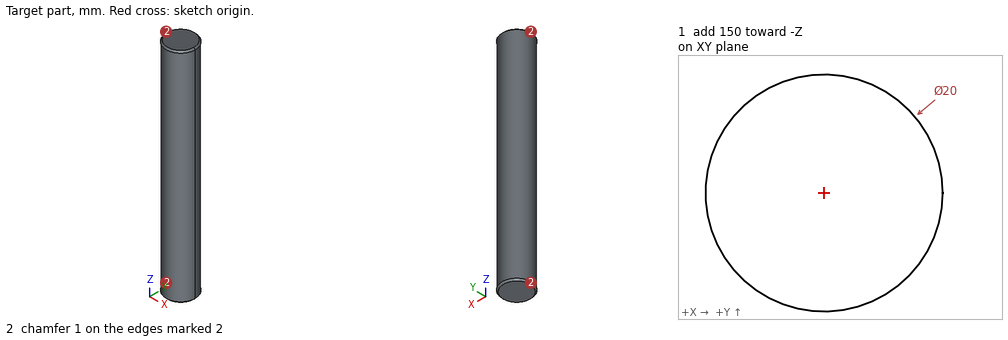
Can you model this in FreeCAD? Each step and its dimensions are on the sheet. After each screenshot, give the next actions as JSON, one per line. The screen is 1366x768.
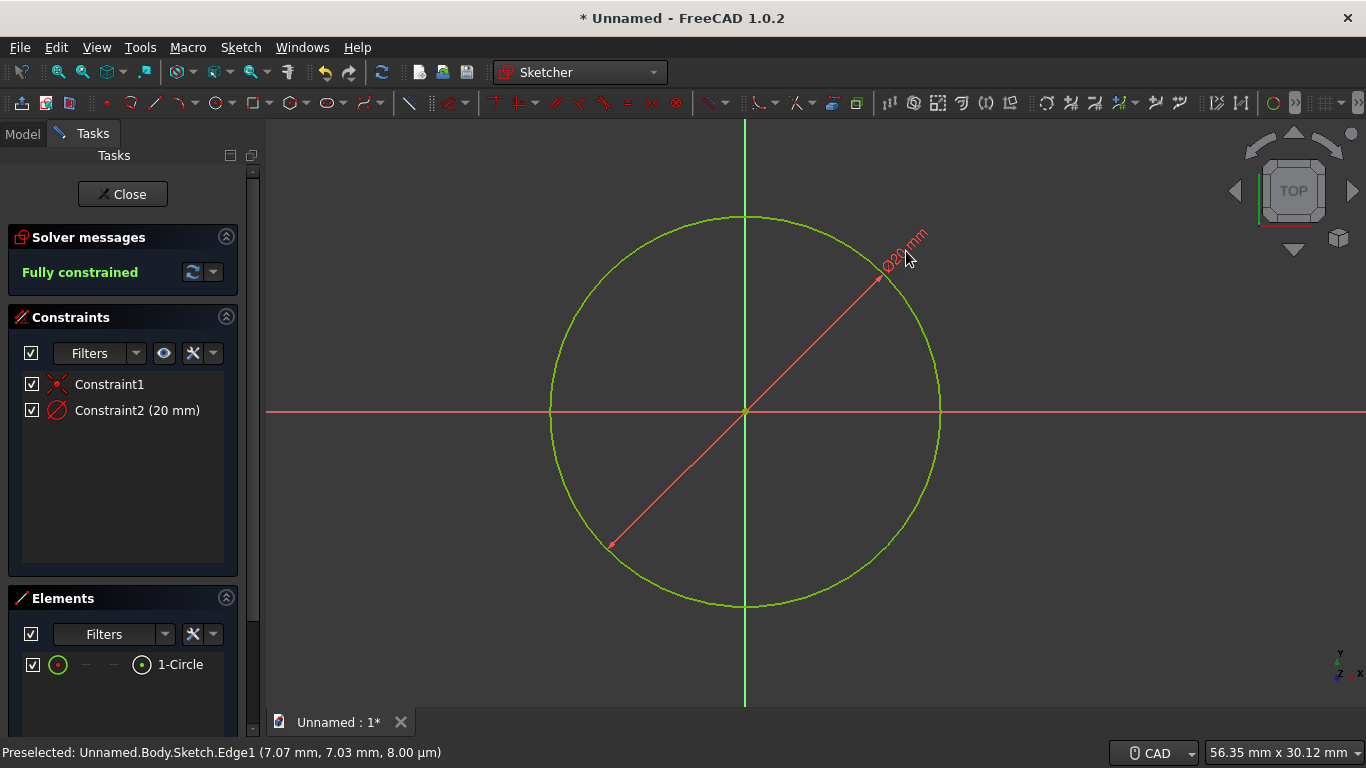
{"action": "left_click", "coordinate": [123, 194]}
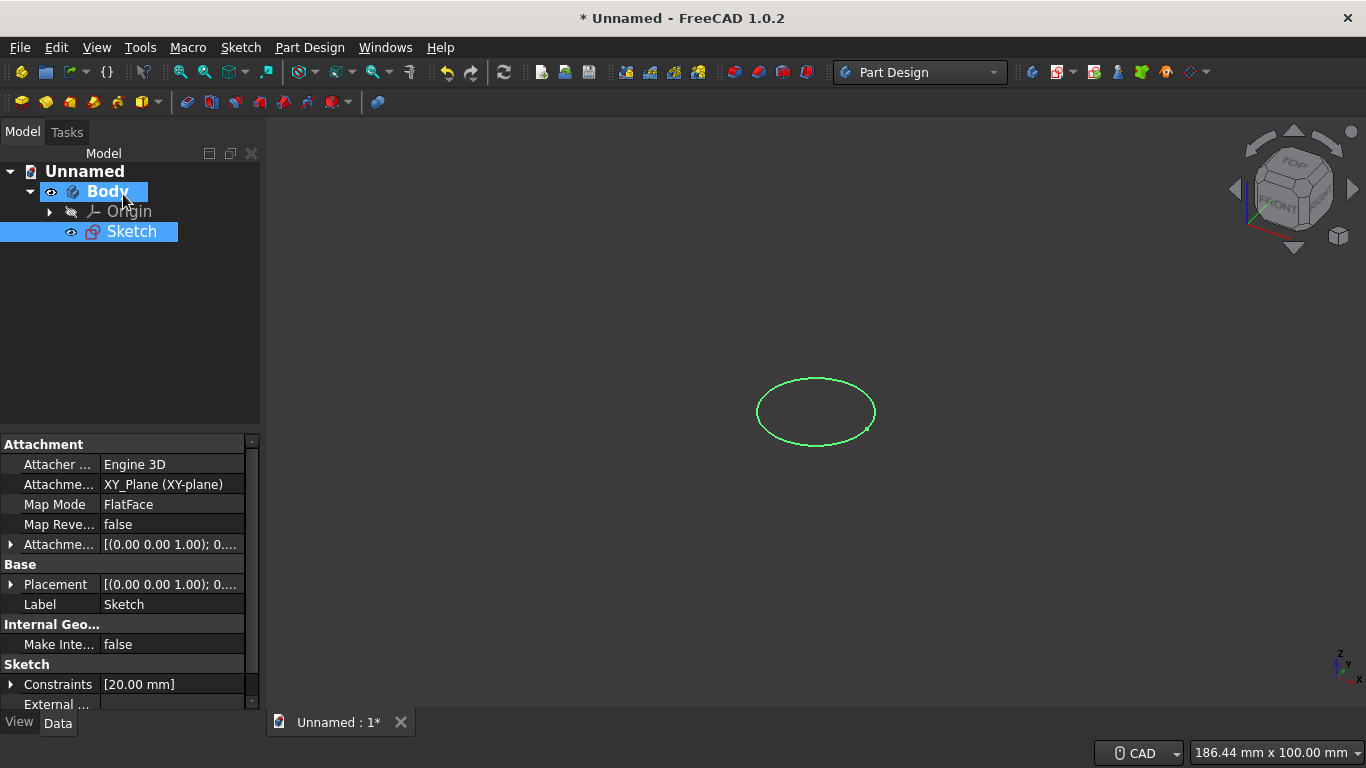
{"action": "left_click", "coordinate": [22, 102]}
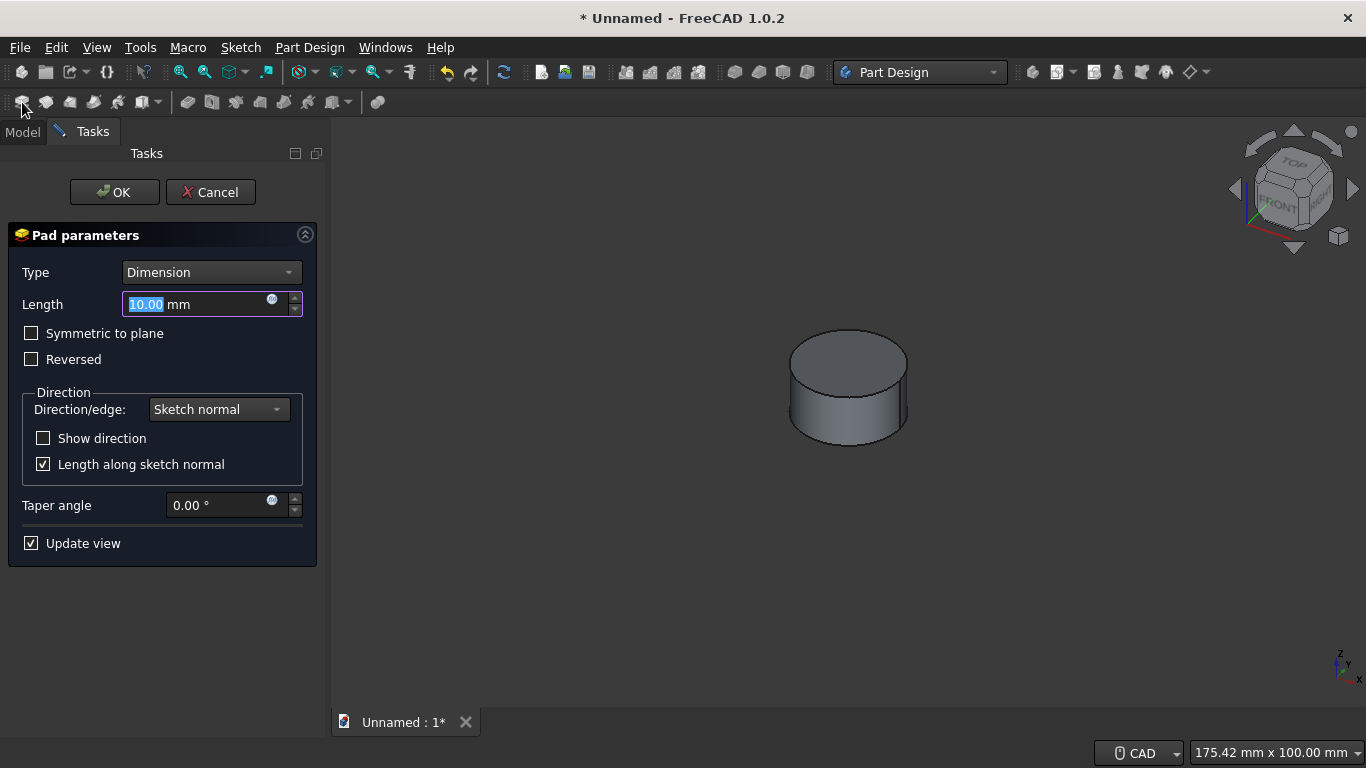
{"action": "type", "text": "150"}
{"action": "key", "text": "Tab"}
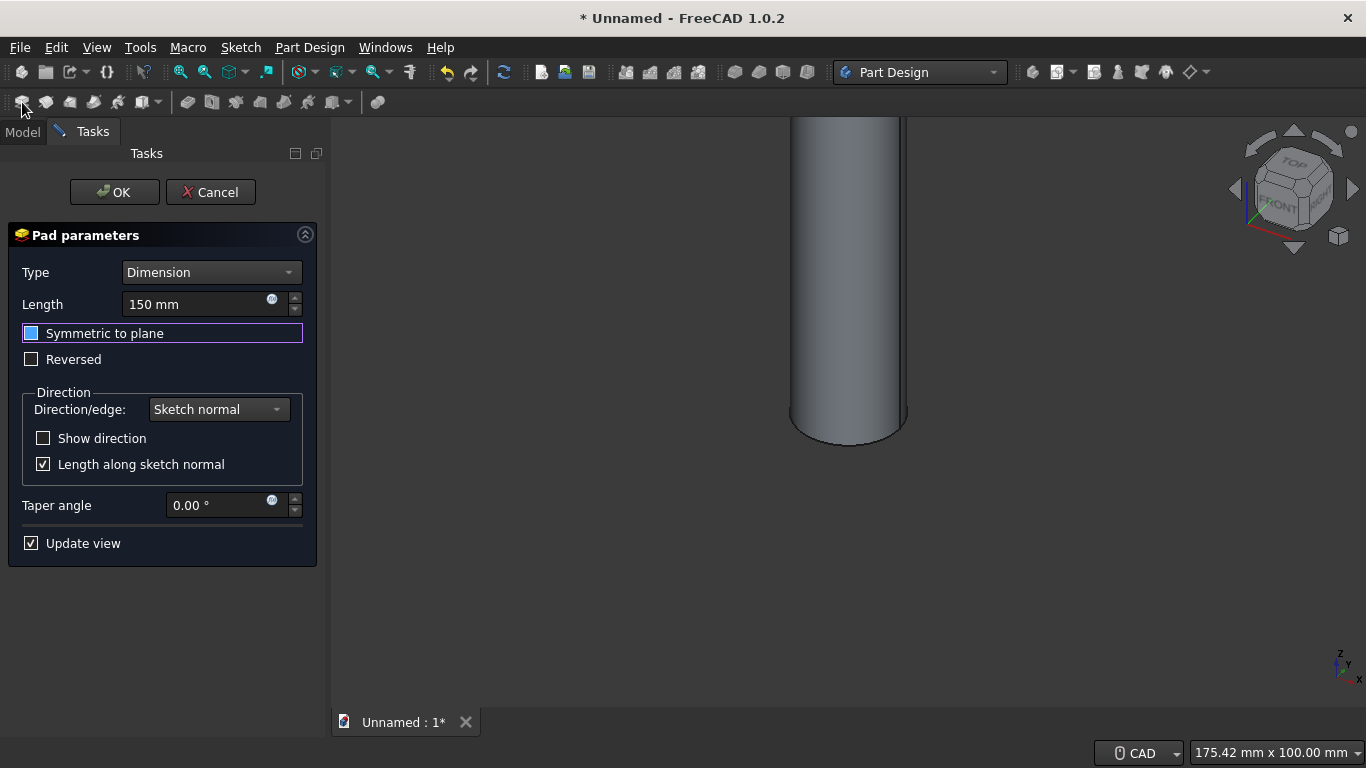
{"action": "left_click", "coordinate": [30, 359]}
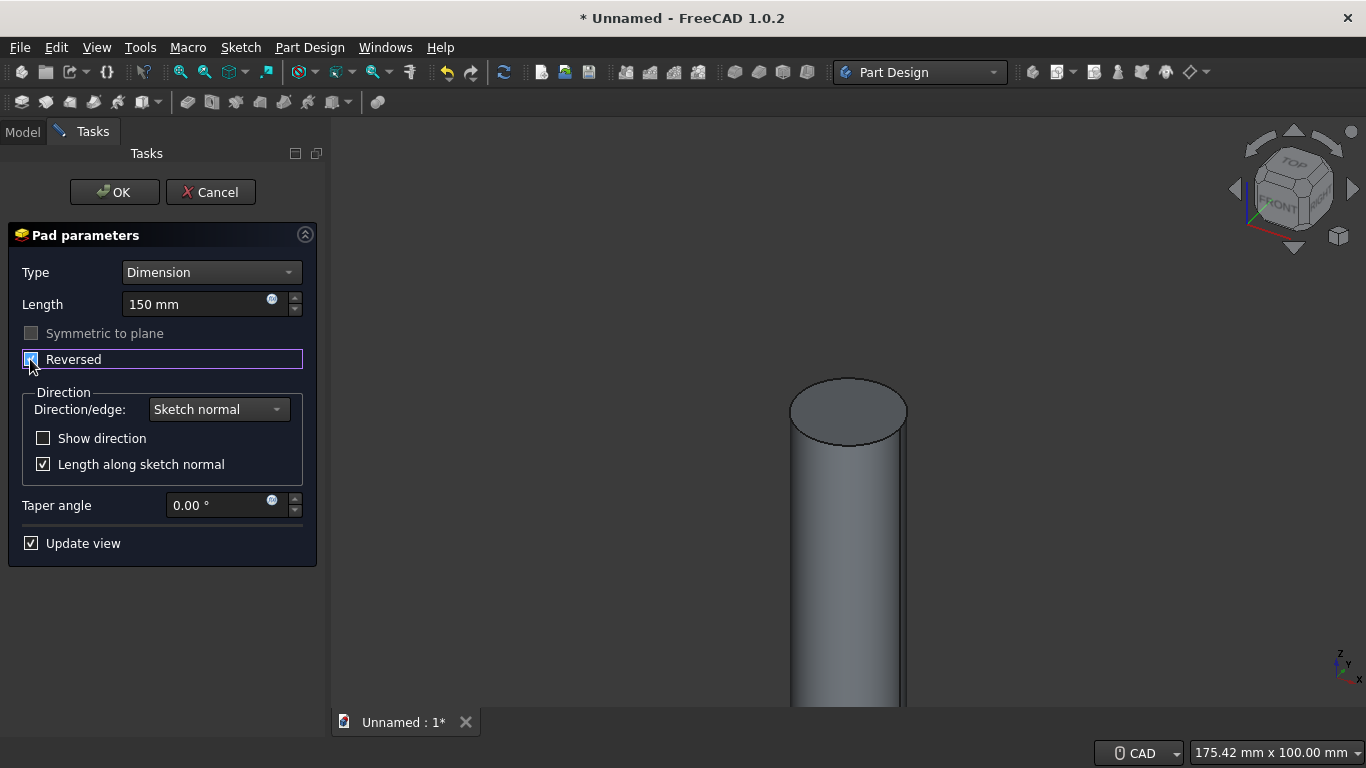
{"action": "left_click", "coordinate": [115, 192]}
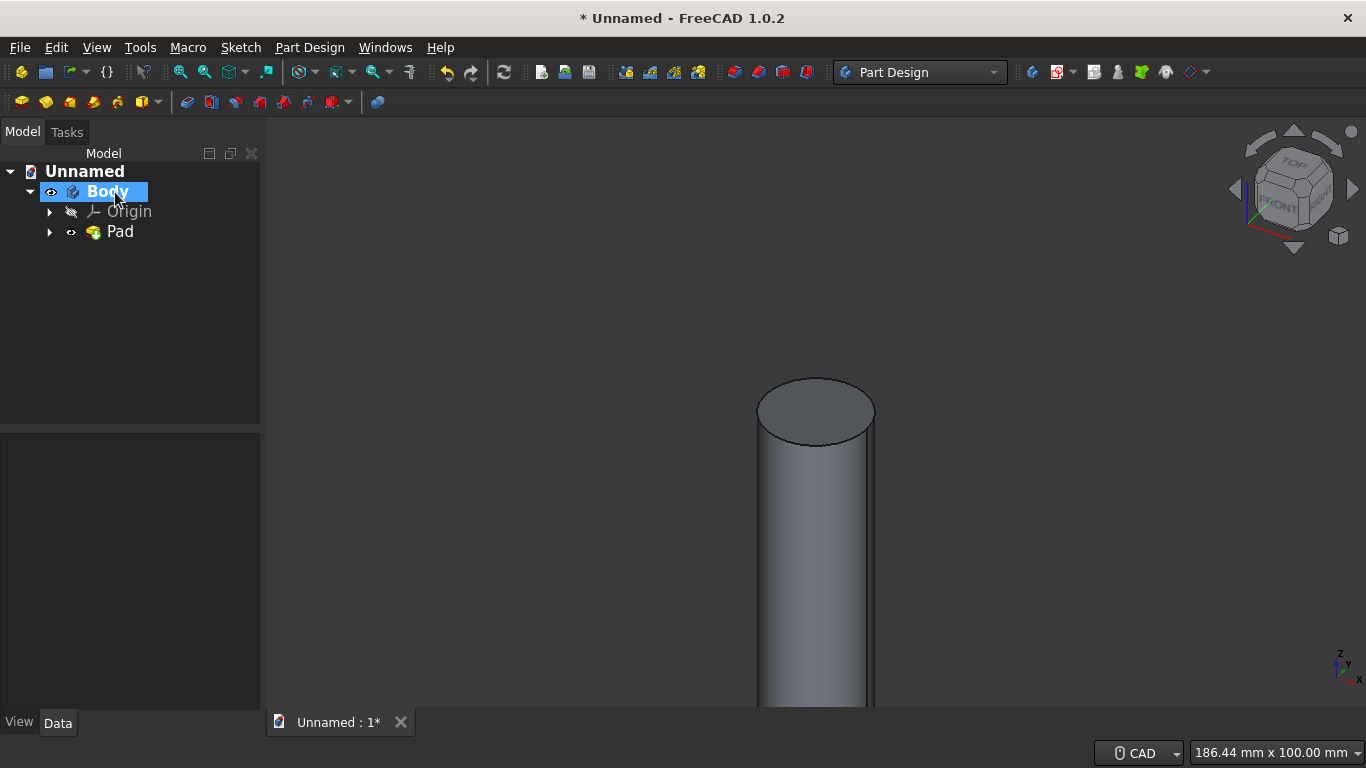
{"action": "key", "text": "v f"}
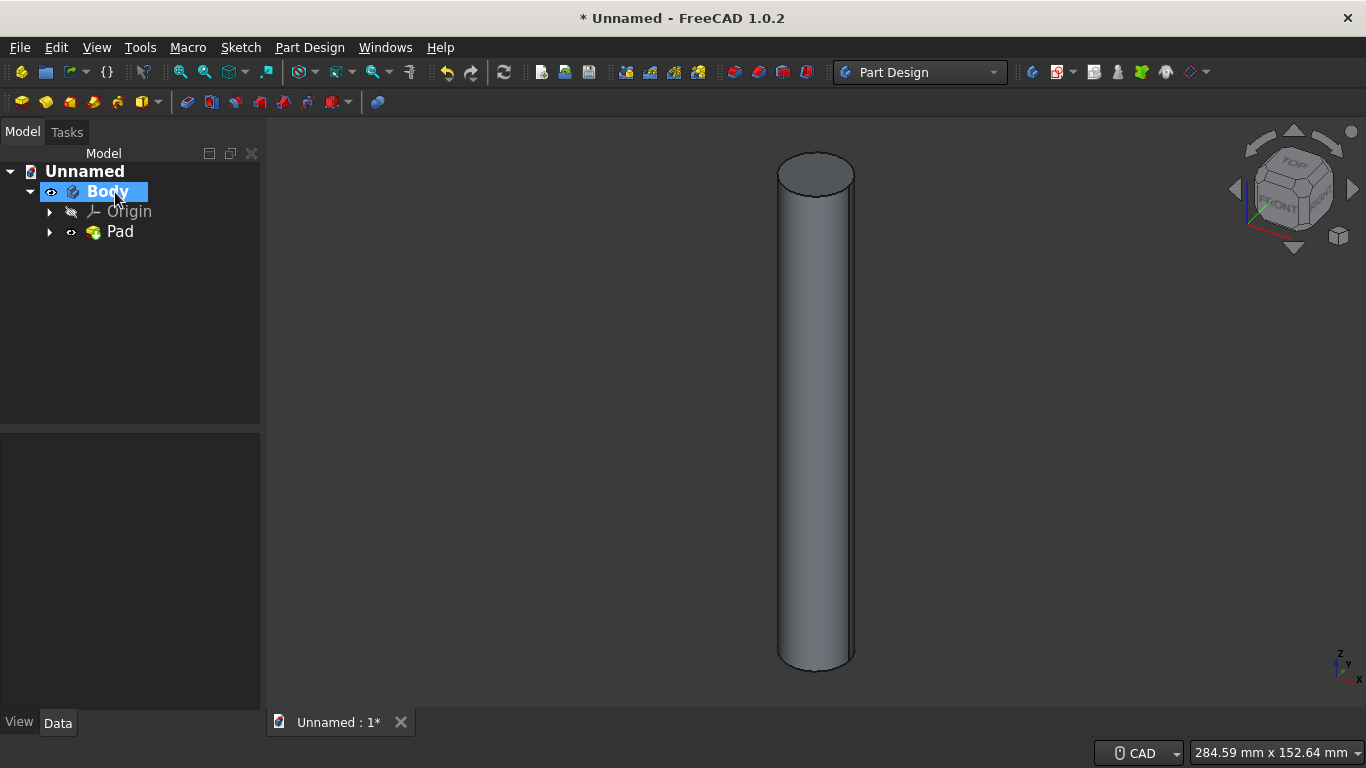
{"action": "left_click", "coordinate": [778, 176]}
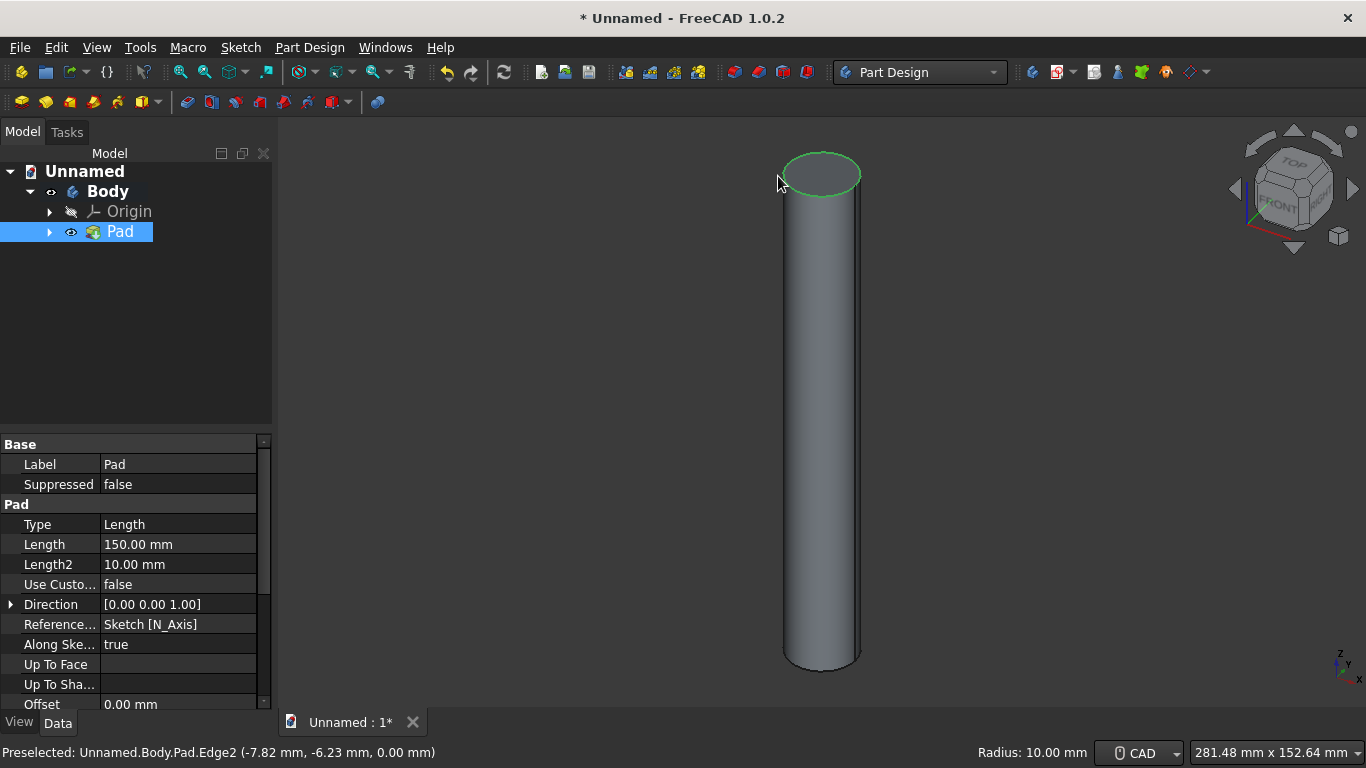
{"action": "key", "text": "0"}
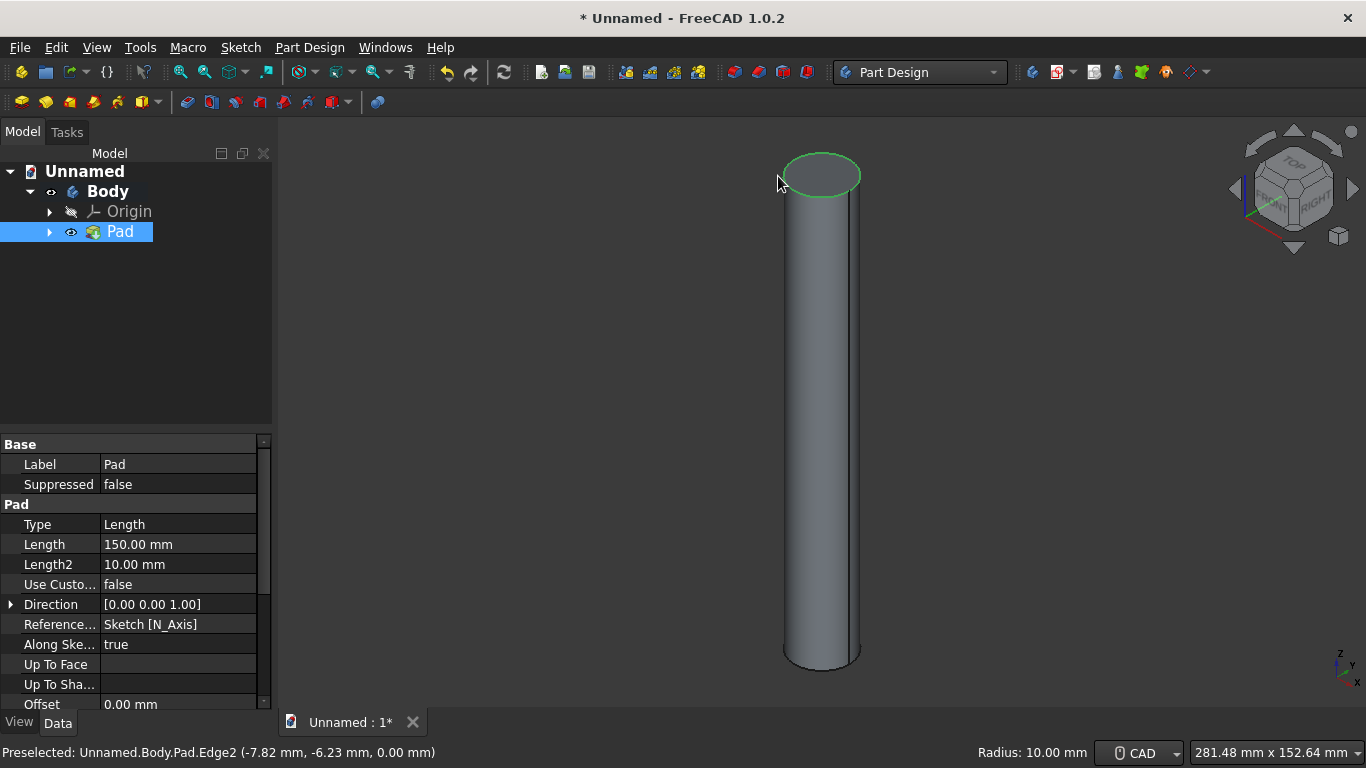
{"action": "key", "text": "2"}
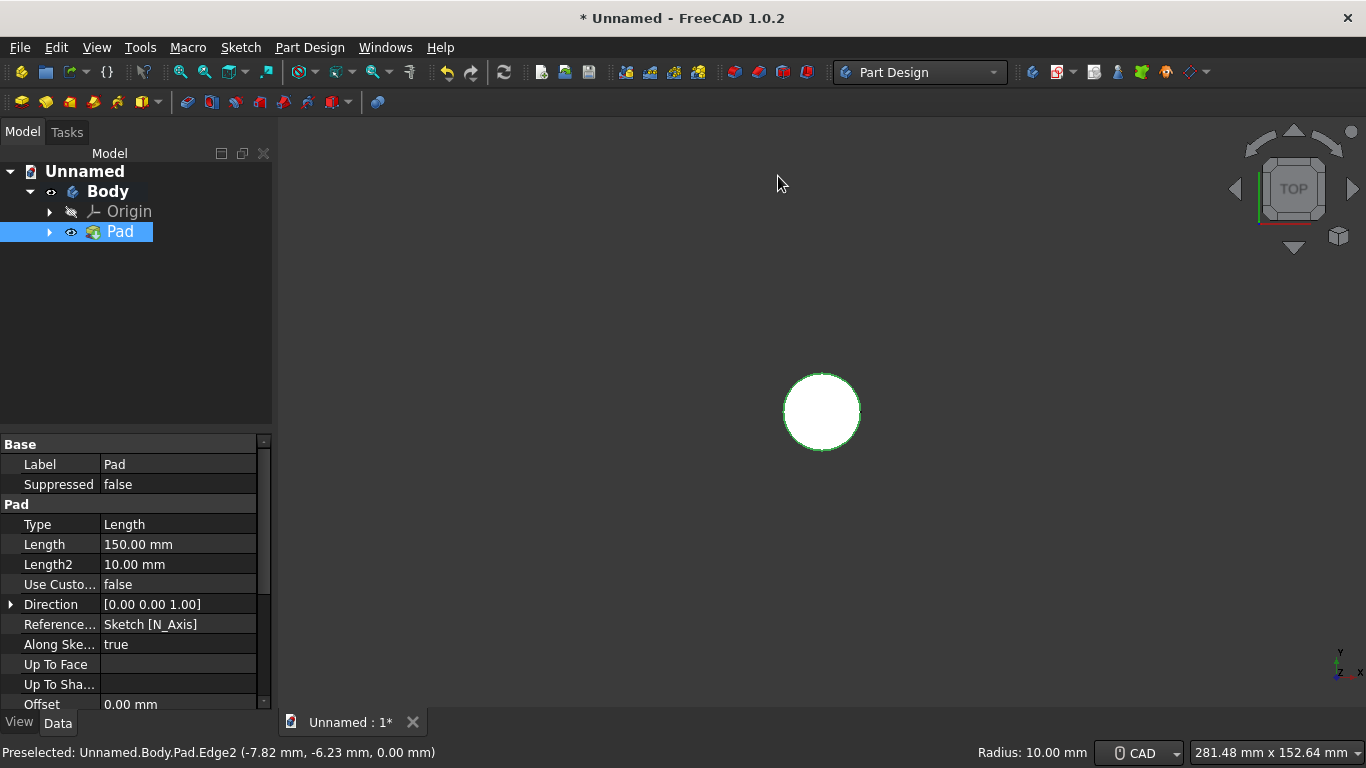
{"action": "left_click", "coordinate": [182, 72]}